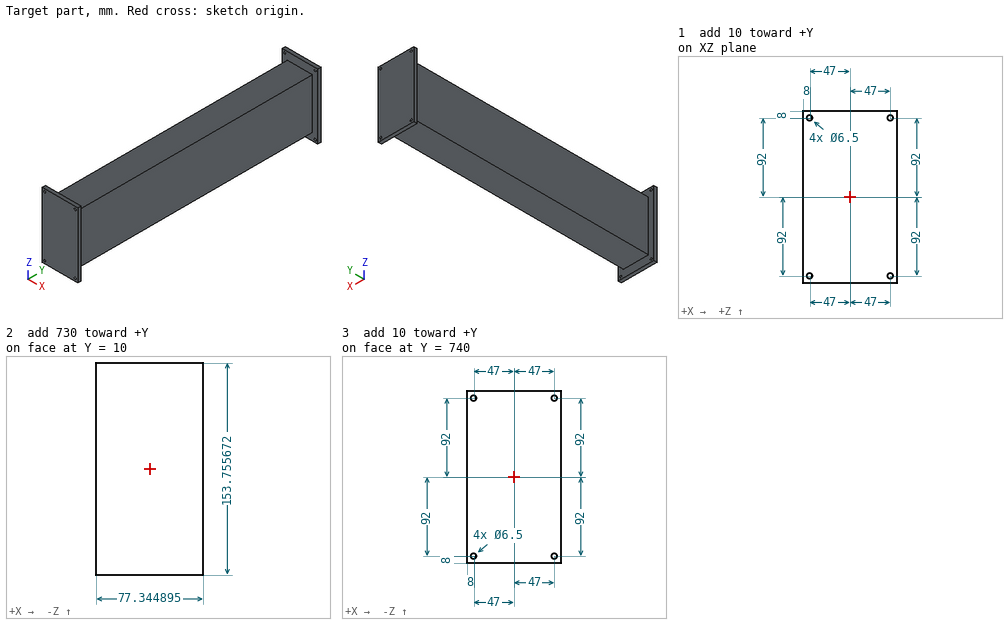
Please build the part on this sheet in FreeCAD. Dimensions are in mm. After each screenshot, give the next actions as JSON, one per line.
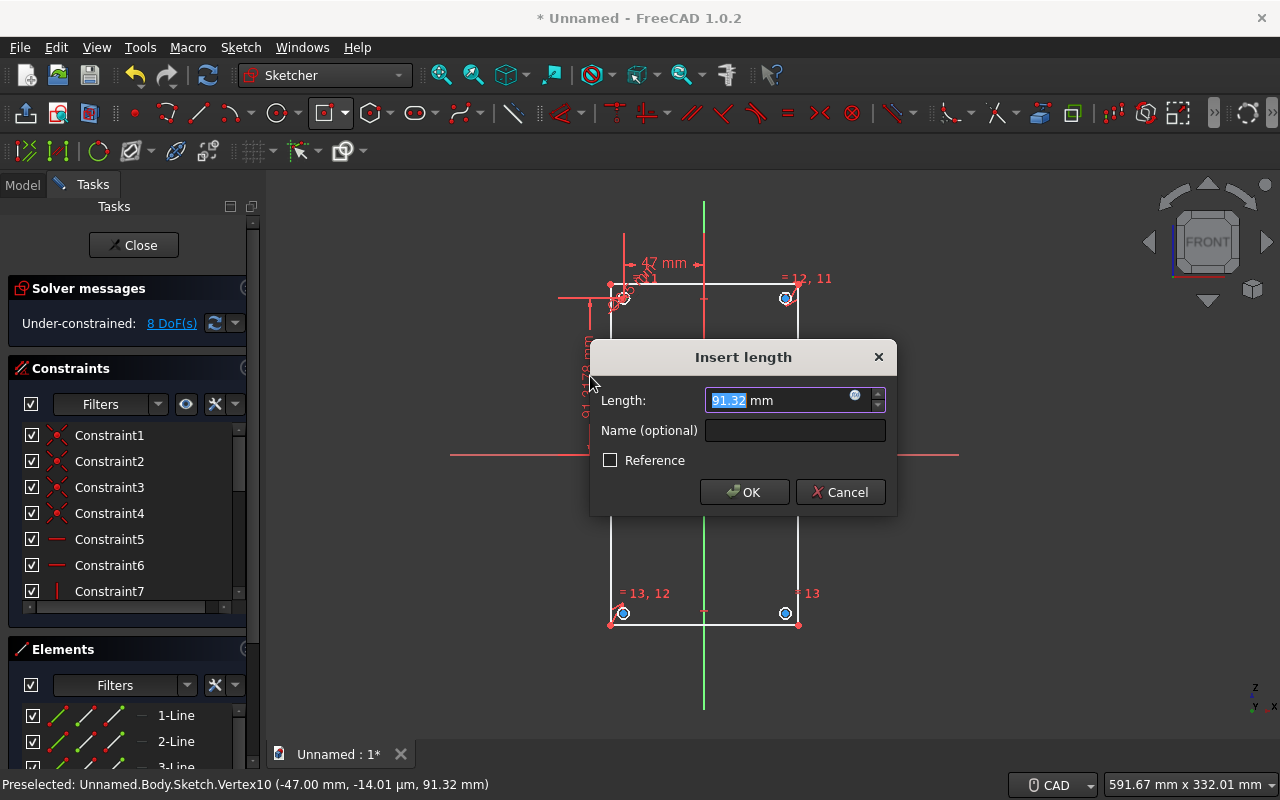
{"action": "type", "text": "92"}
{"action": "key", "text": "Return"}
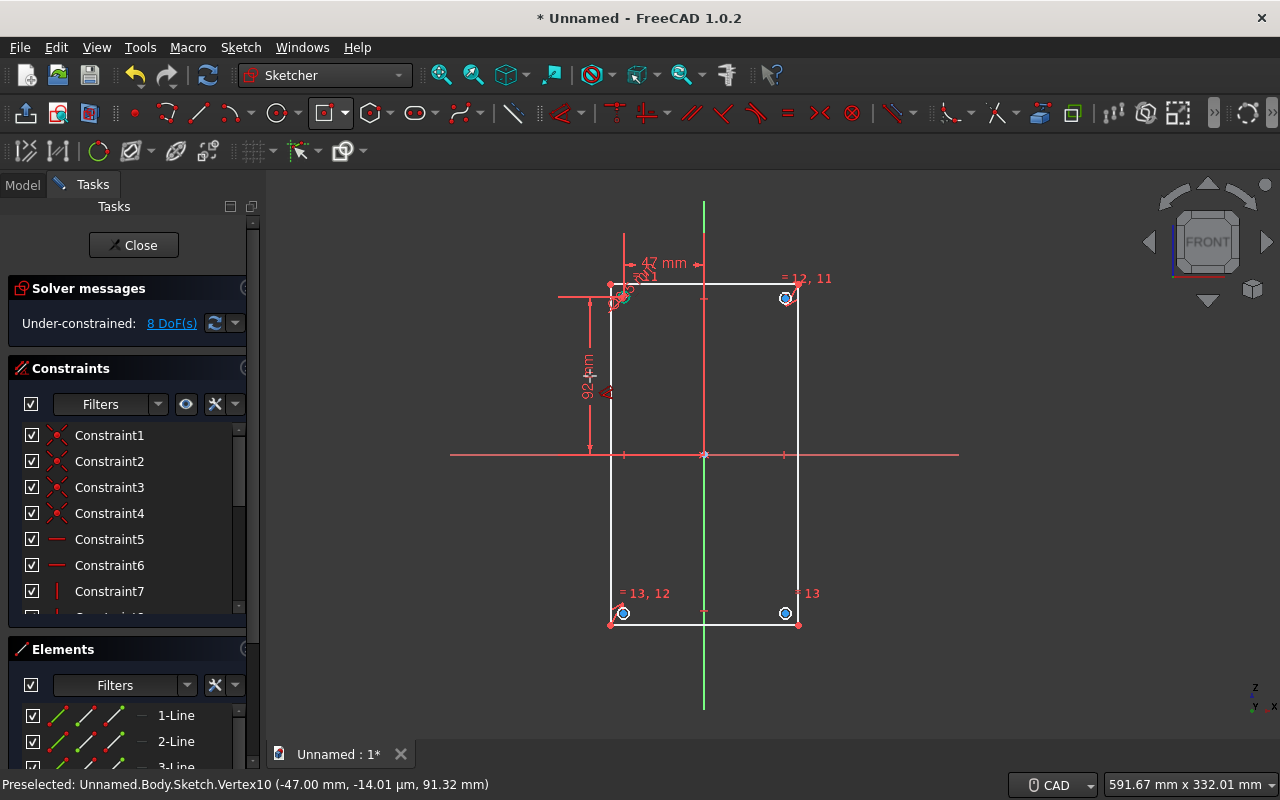
{"action": "left_click", "coordinate": [785, 298]}
{"action": "left_click", "coordinate": [745, 264]}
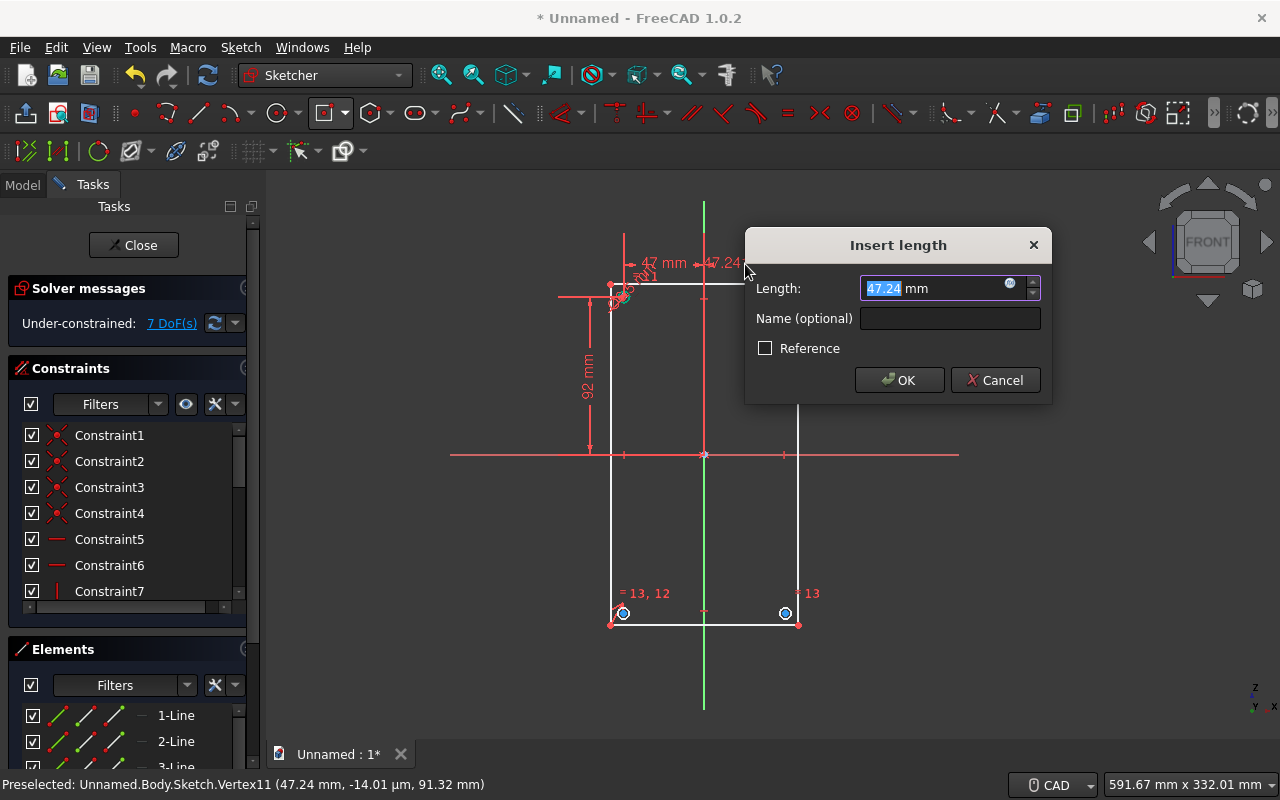
{"action": "type", "text": "47"}
{"action": "key", "text": "Return"}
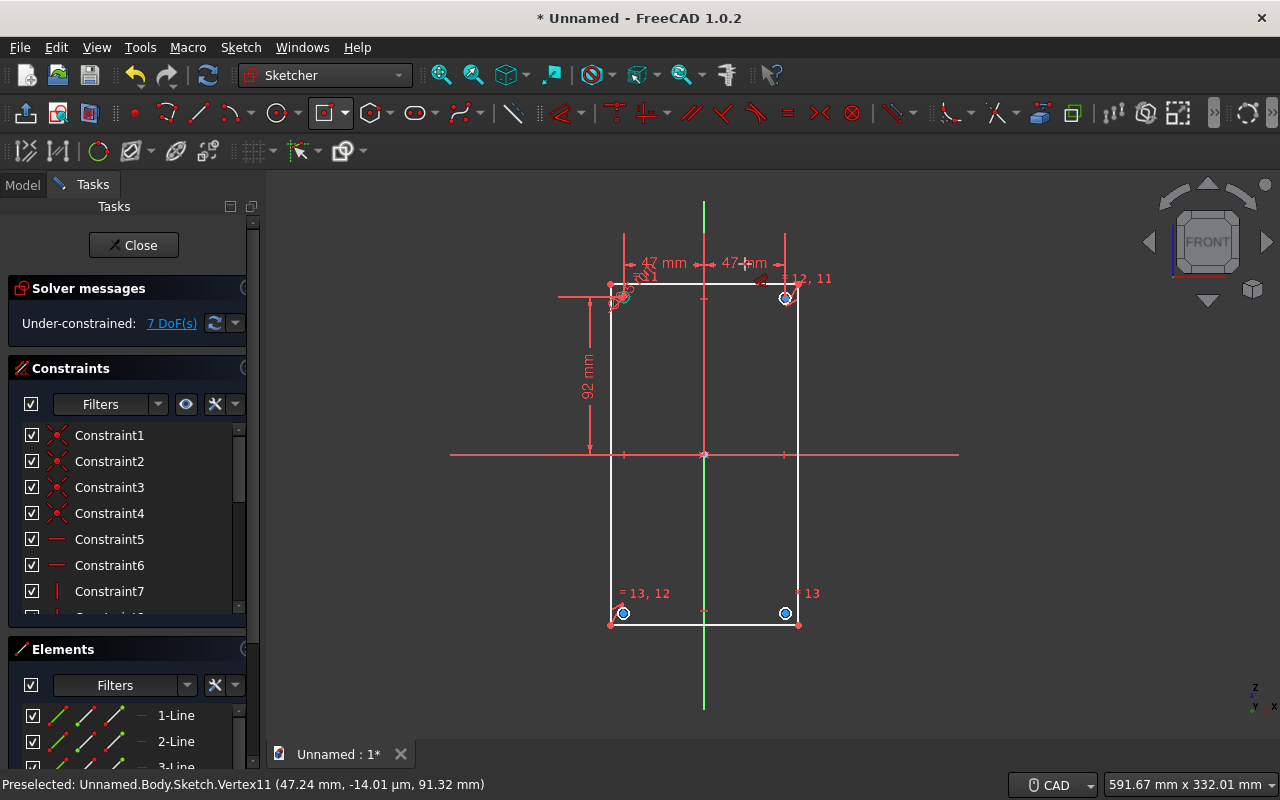
{"action": "left_click", "coordinate": [785, 298]}
{"action": "left_click", "coordinate": [819, 376]}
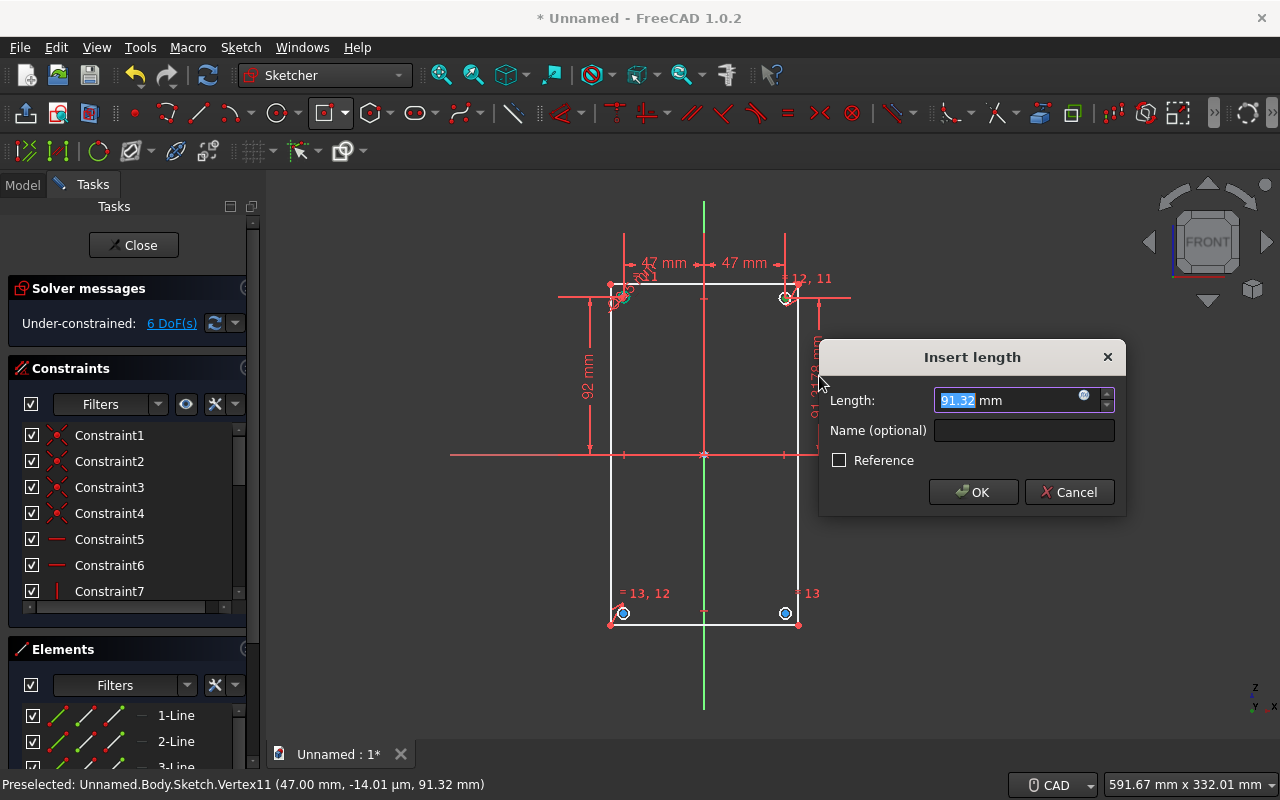
{"action": "type", "text": "92"}
{"action": "key", "text": "Return"}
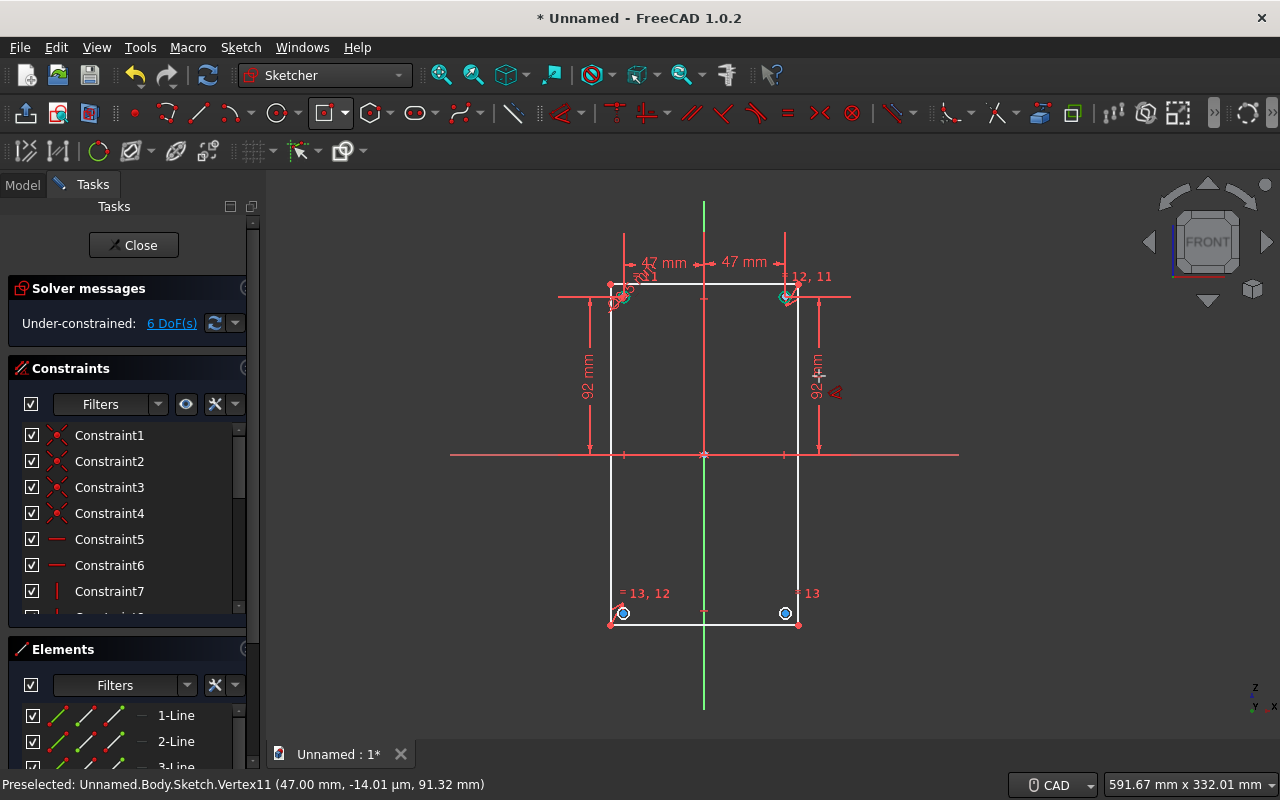
{"action": "left_click", "coordinate": [623, 613]}
{"action": "left_click", "coordinate": [664, 647]}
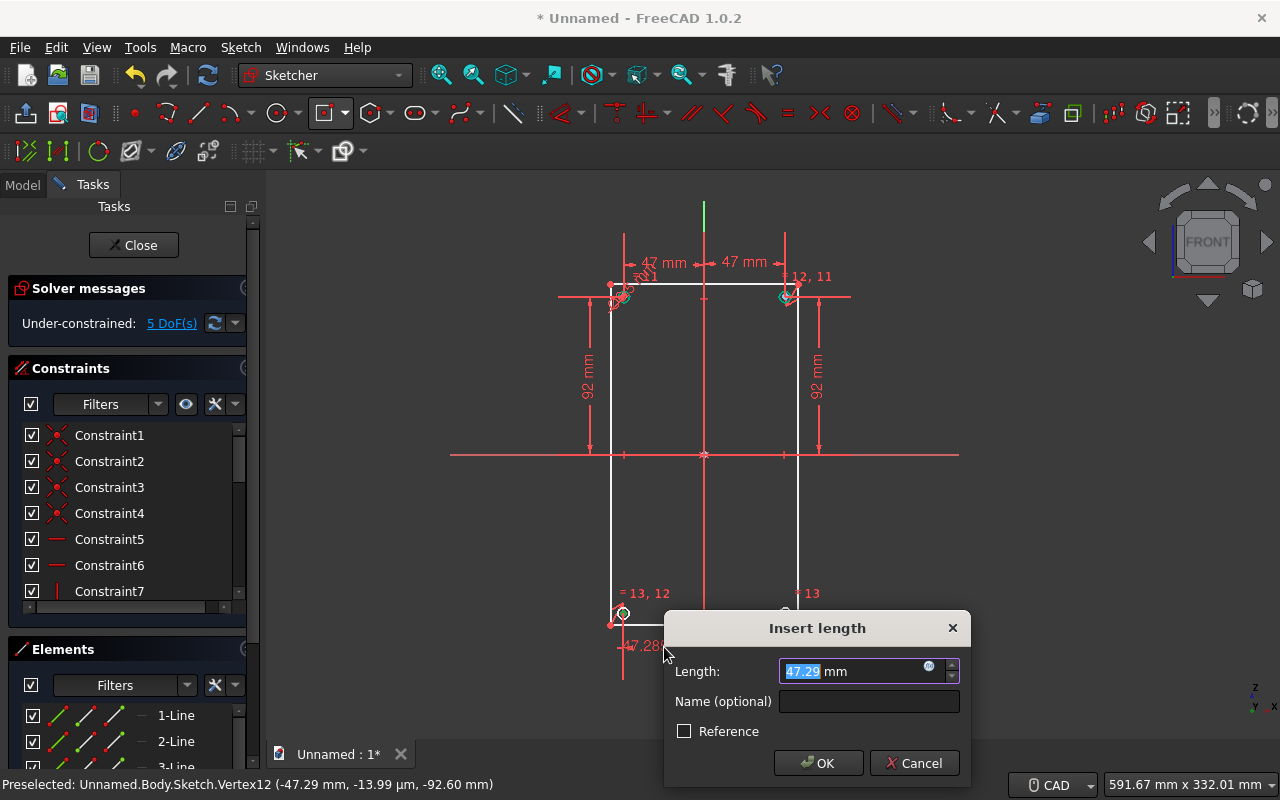
{"action": "type", "text": "47"}
{"action": "key", "text": "Return"}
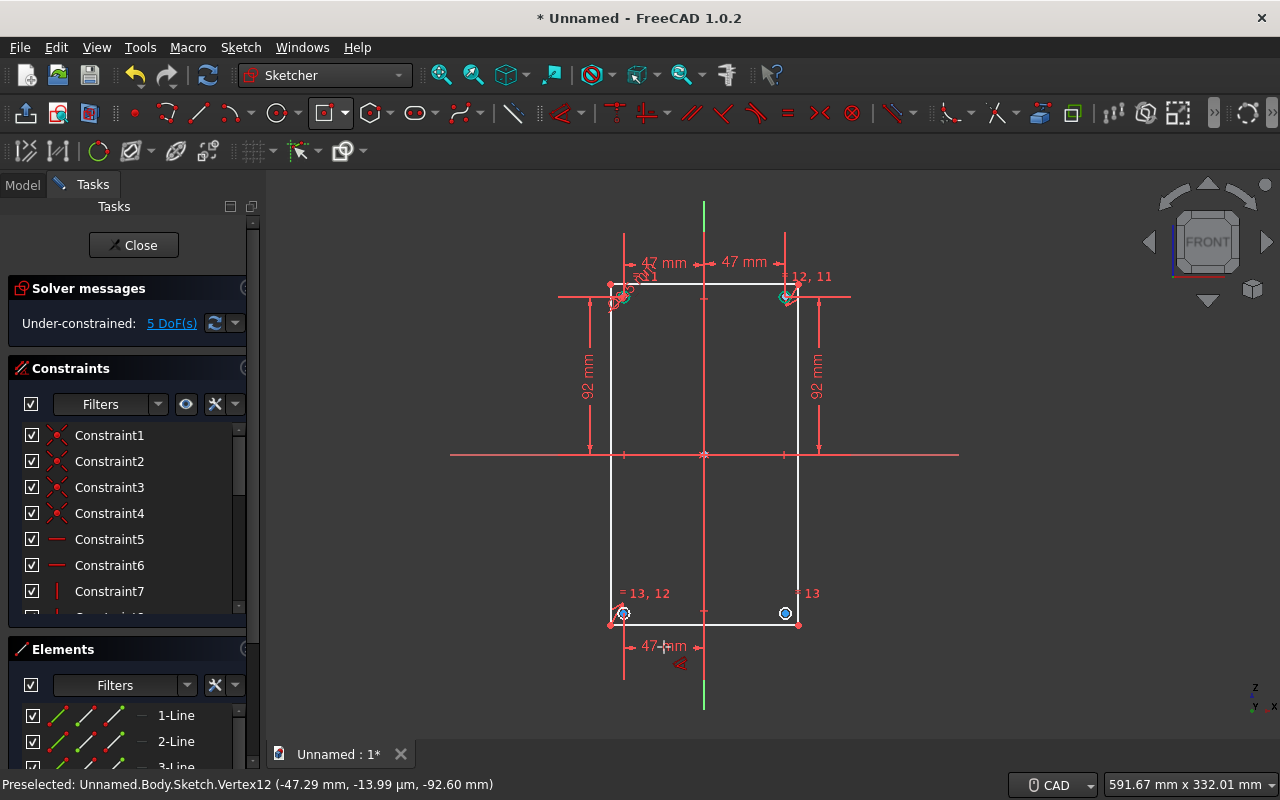
{"action": "left_click", "coordinate": [624, 613]}
{"action": "left_click", "coordinate": [590, 534]}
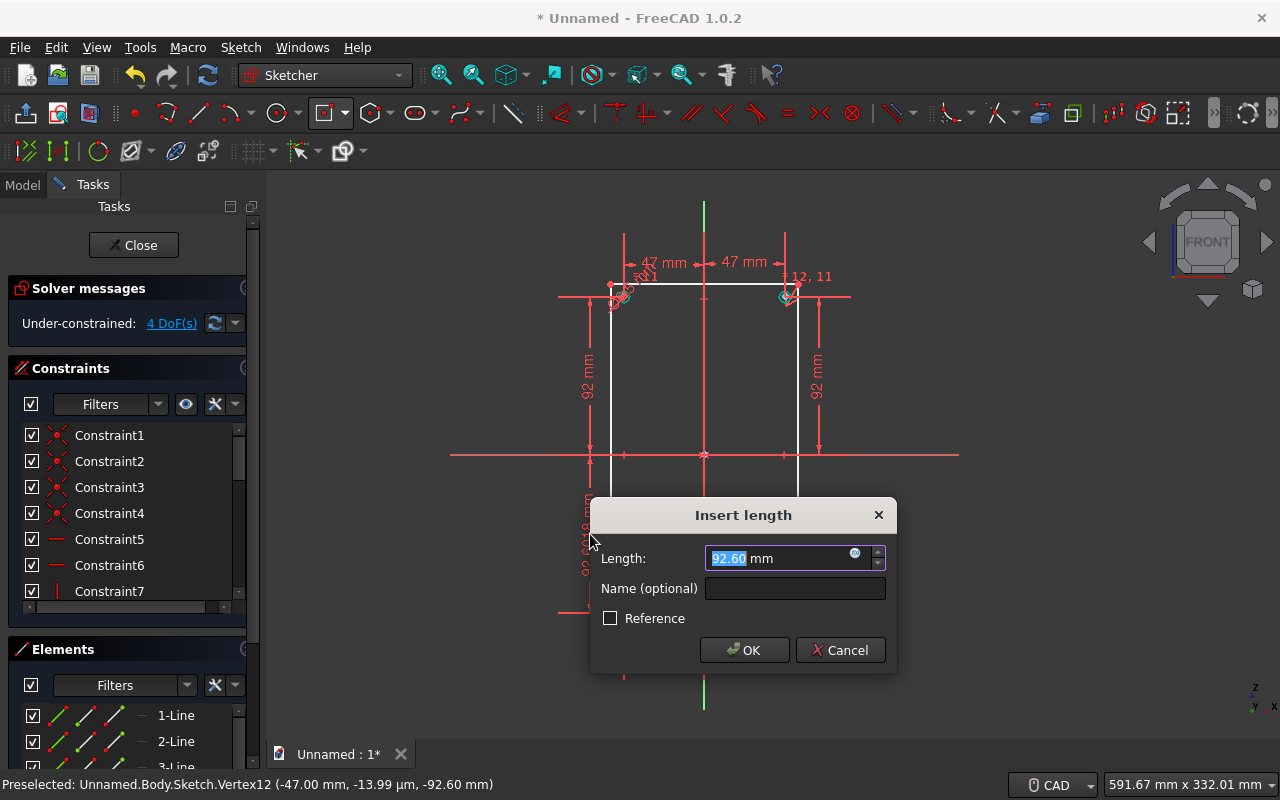
{"action": "type", "text": "92"}
{"action": "key", "text": "Return"}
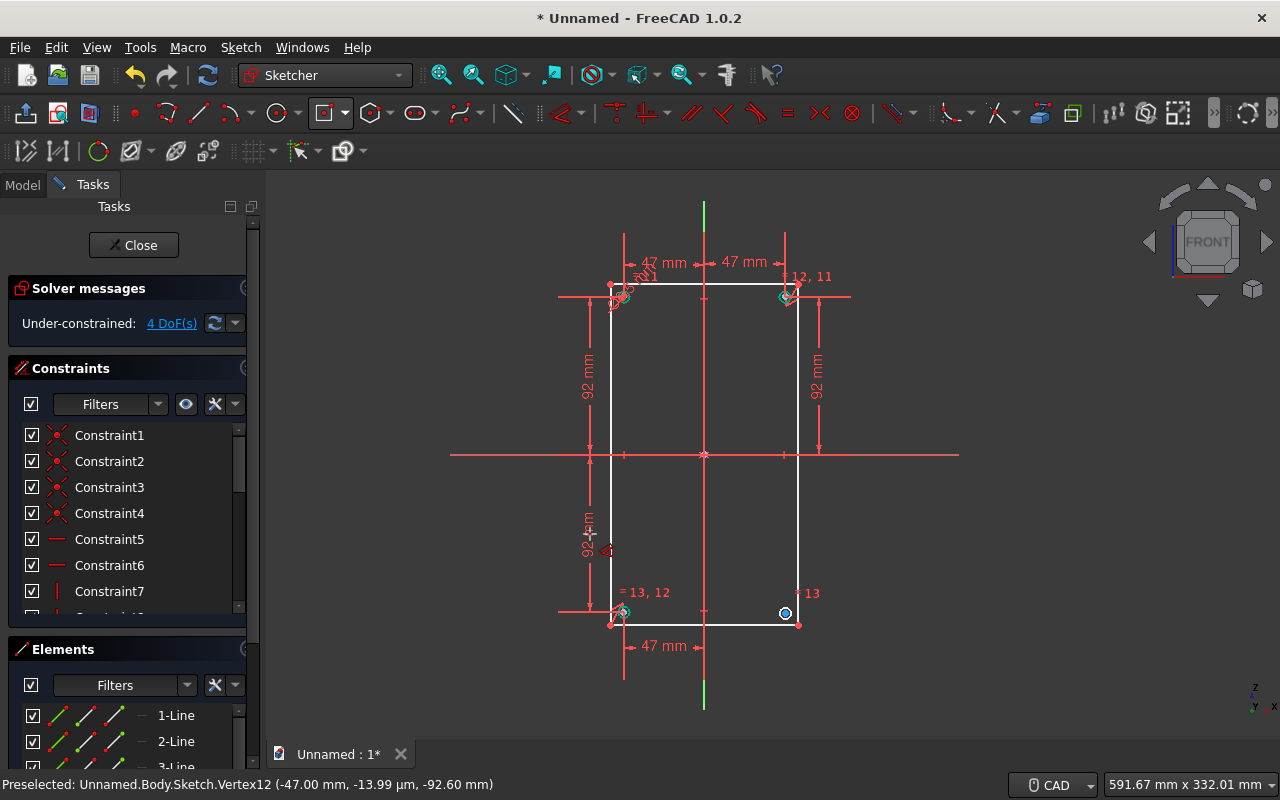
{"action": "left_click", "coordinate": [785, 613]}
{"action": "left_click", "coordinate": [745, 647]}